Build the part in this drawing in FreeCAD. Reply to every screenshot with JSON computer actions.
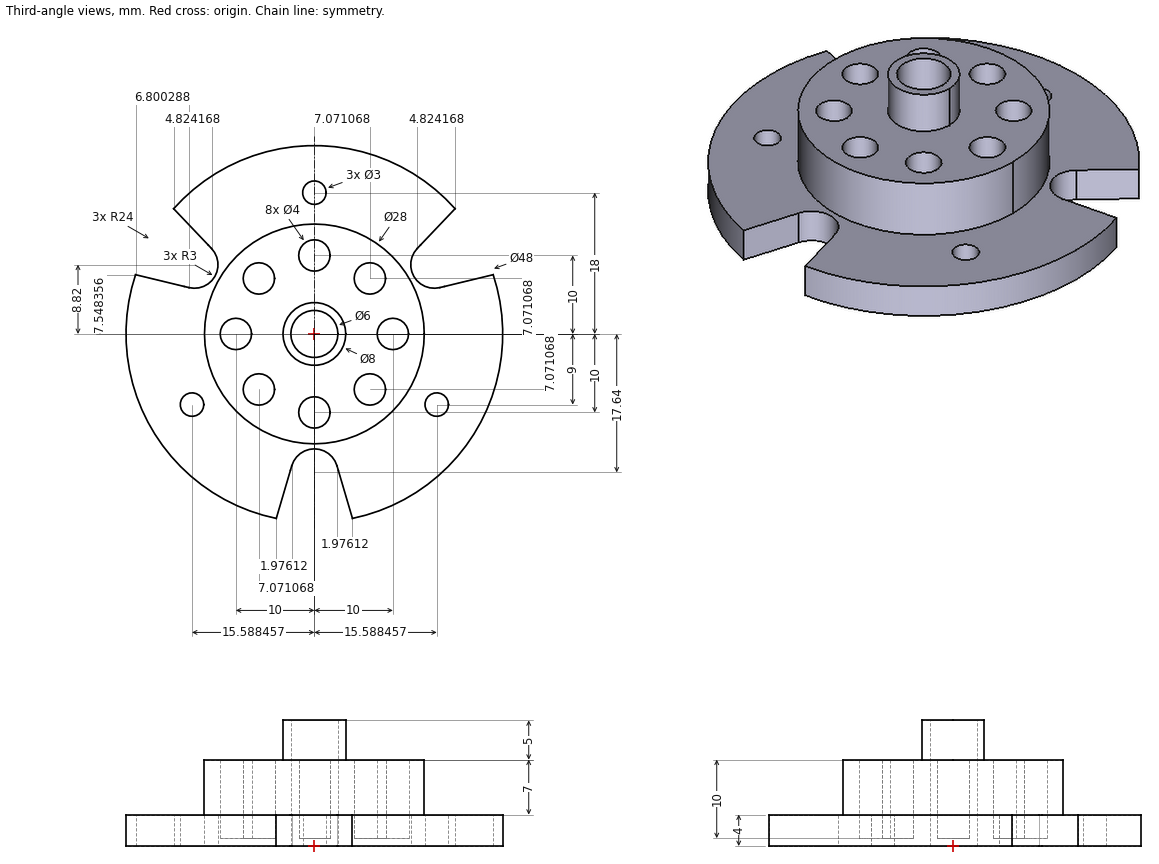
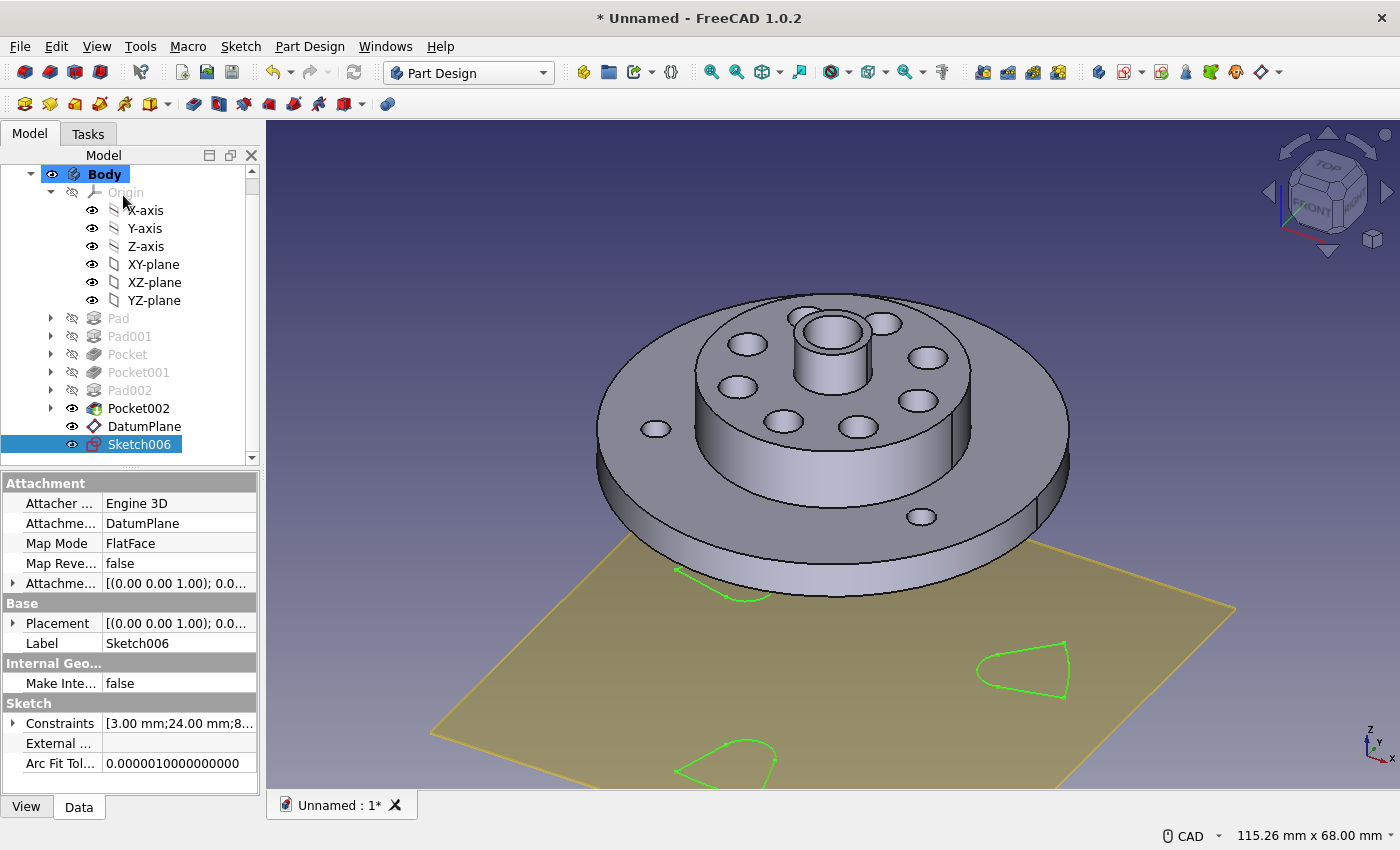
{"action": "left_click", "coordinate": [194, 104]}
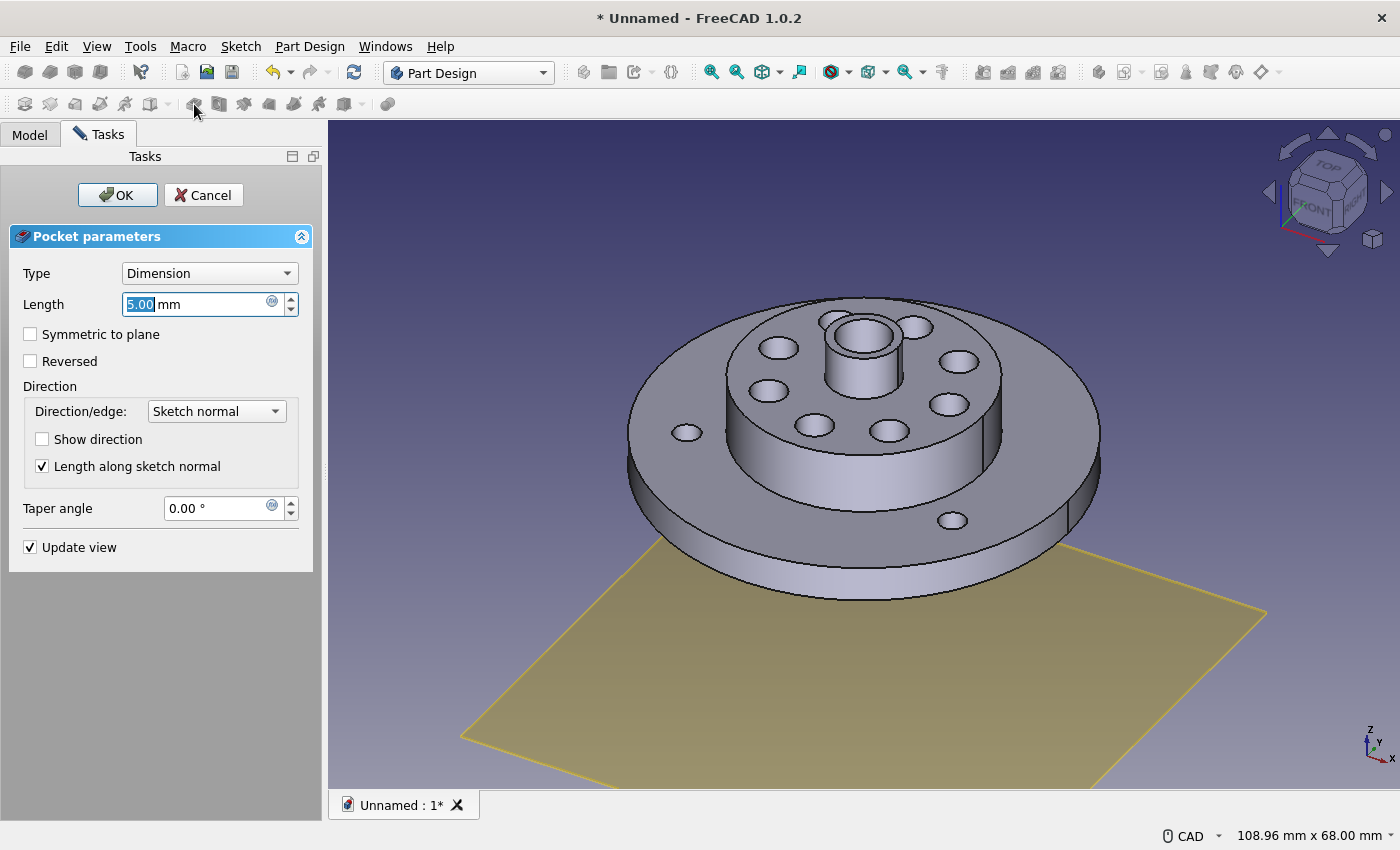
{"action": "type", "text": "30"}
{"action": "key", "text": "Tab"}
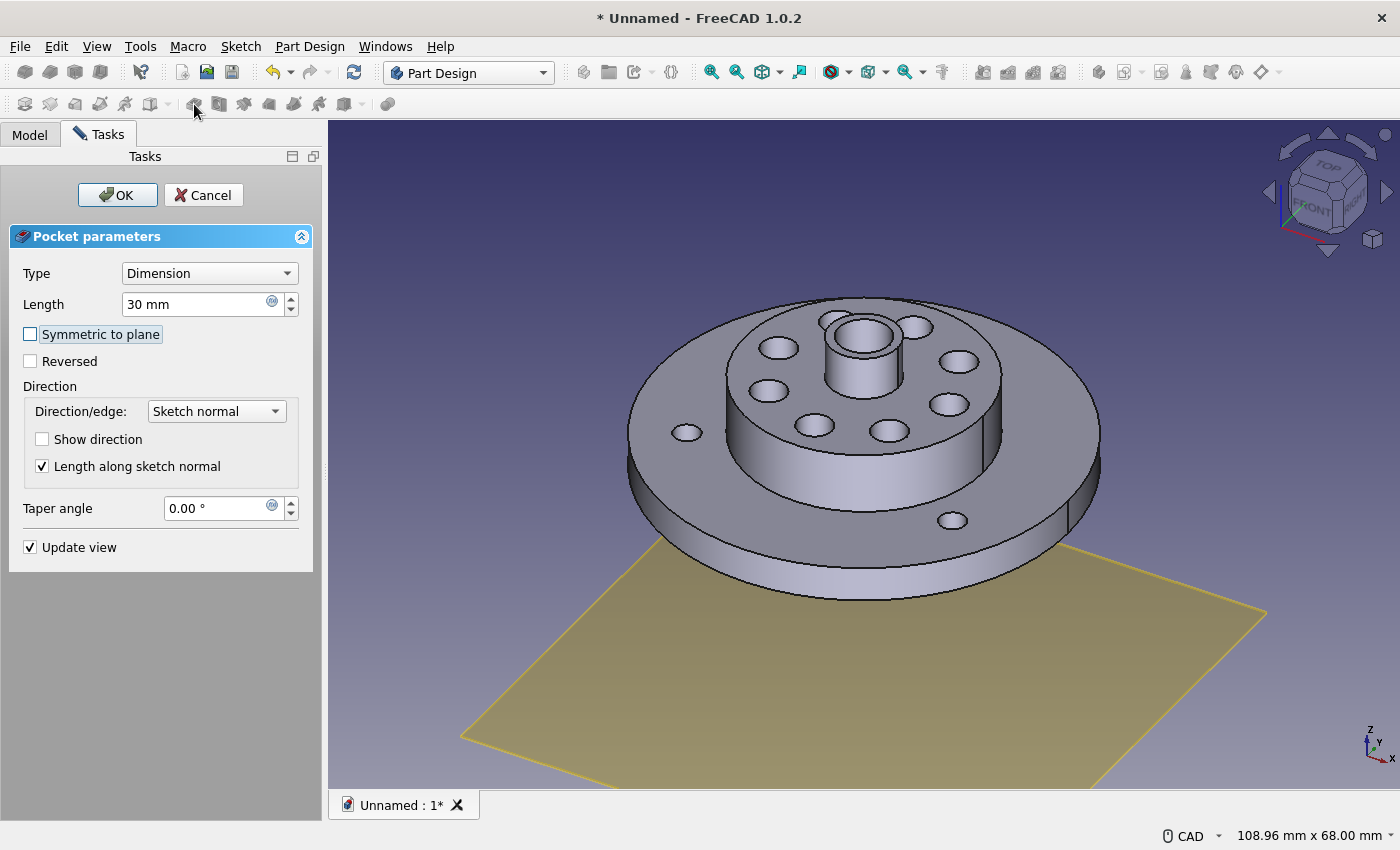
{"action": "left_click", "coordinate": [31, 361]}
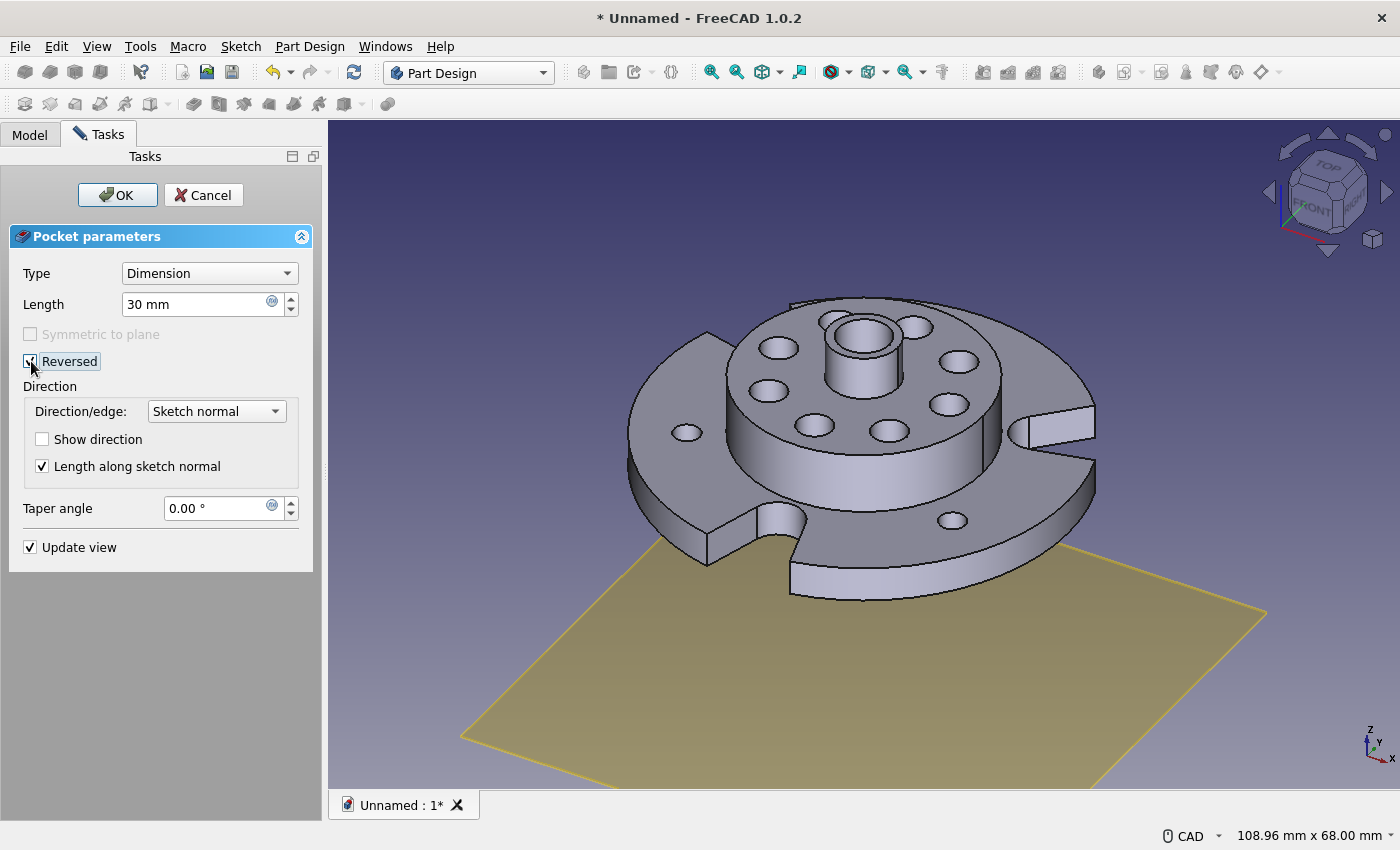
{"action": "left_click", "coordinate": [118, 195]}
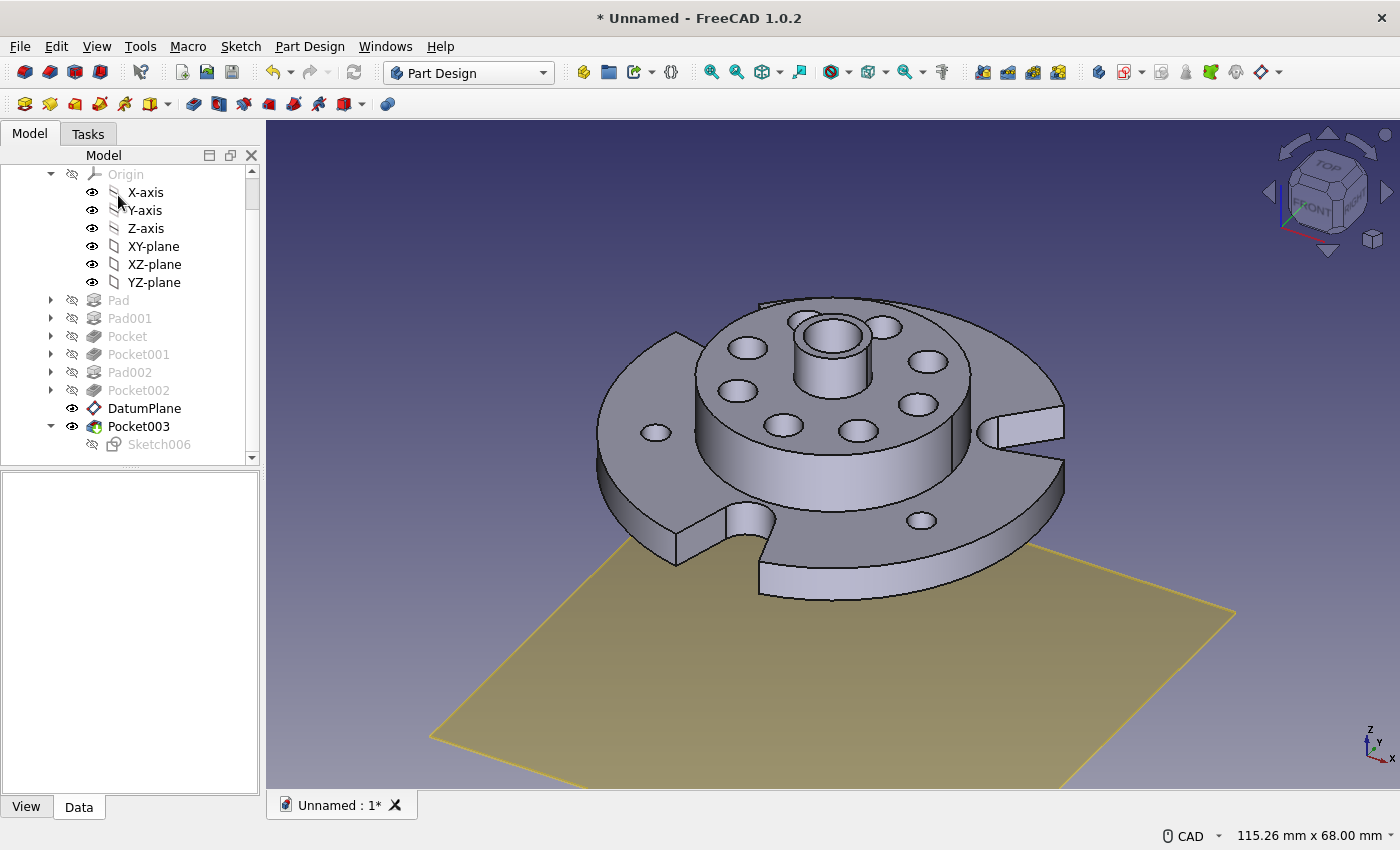
{"action": "left_click", "coordinate": [117, 408]}
{"action": "key", "text": "space"}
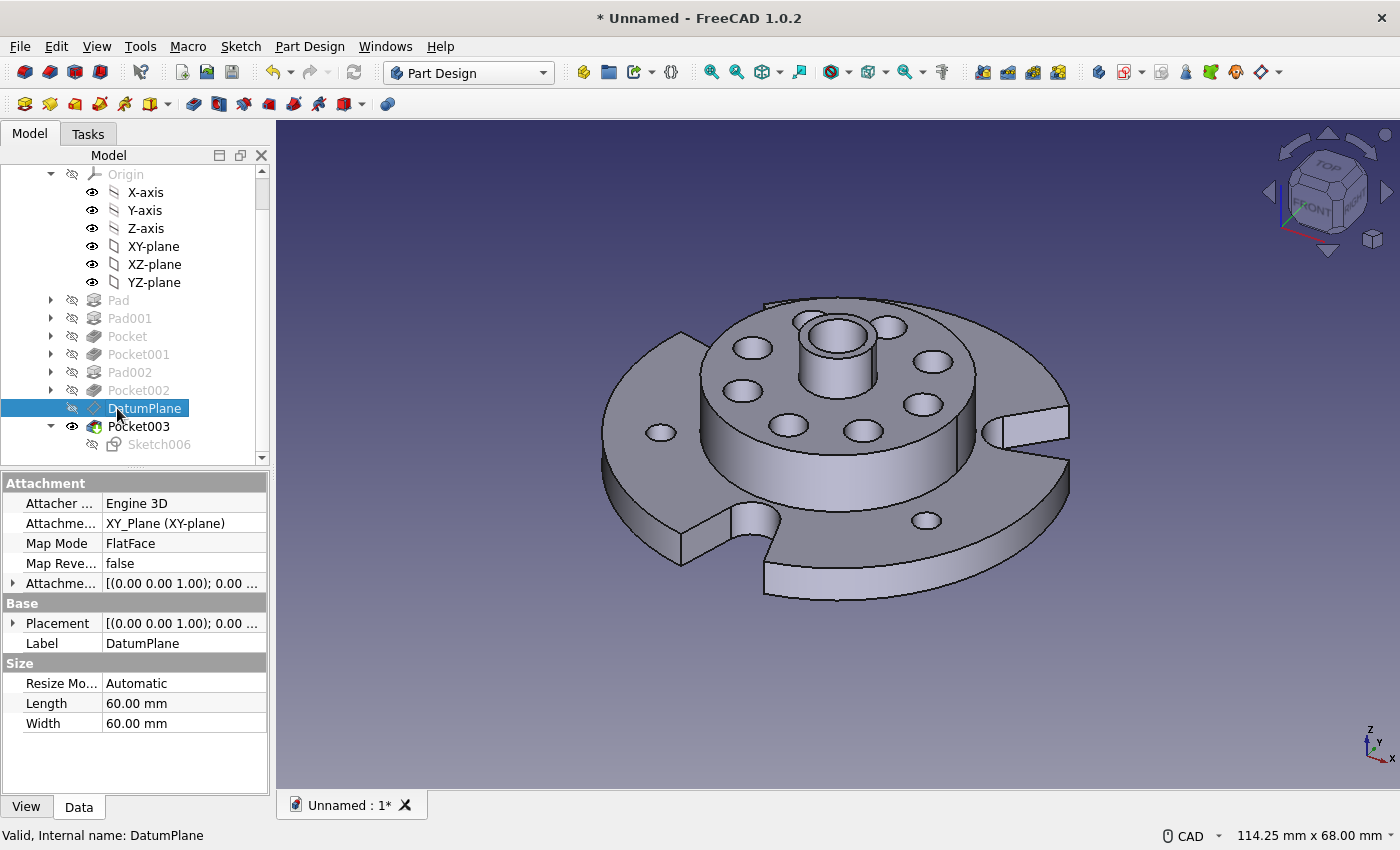
{"action": "key", "text": "0"}